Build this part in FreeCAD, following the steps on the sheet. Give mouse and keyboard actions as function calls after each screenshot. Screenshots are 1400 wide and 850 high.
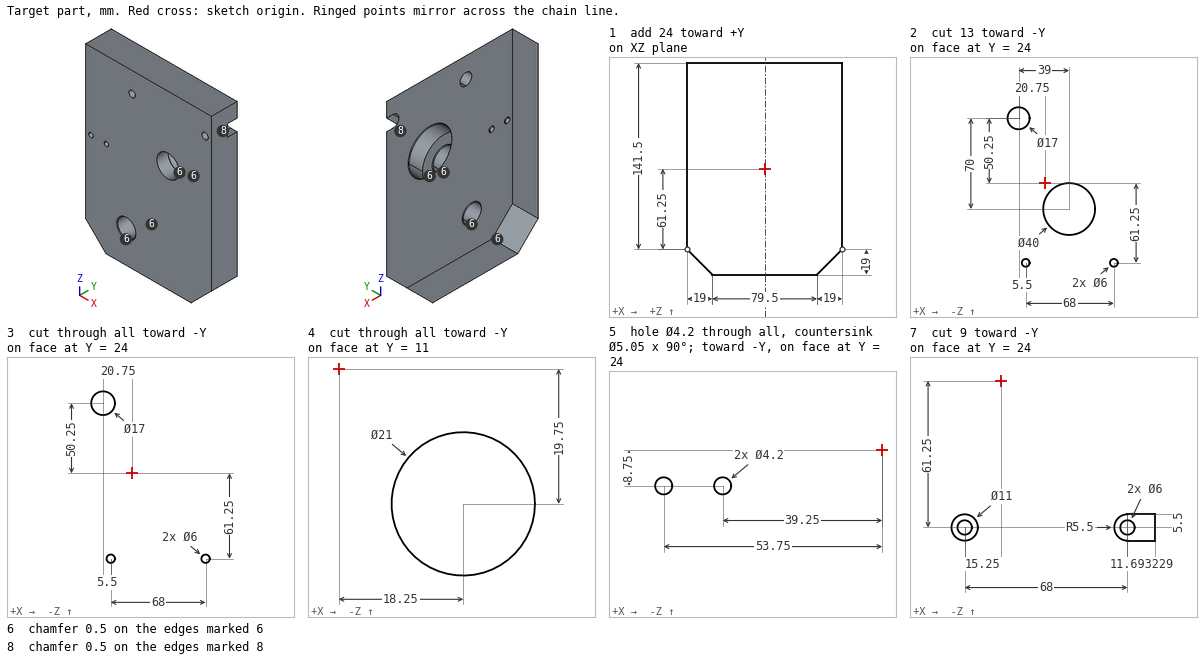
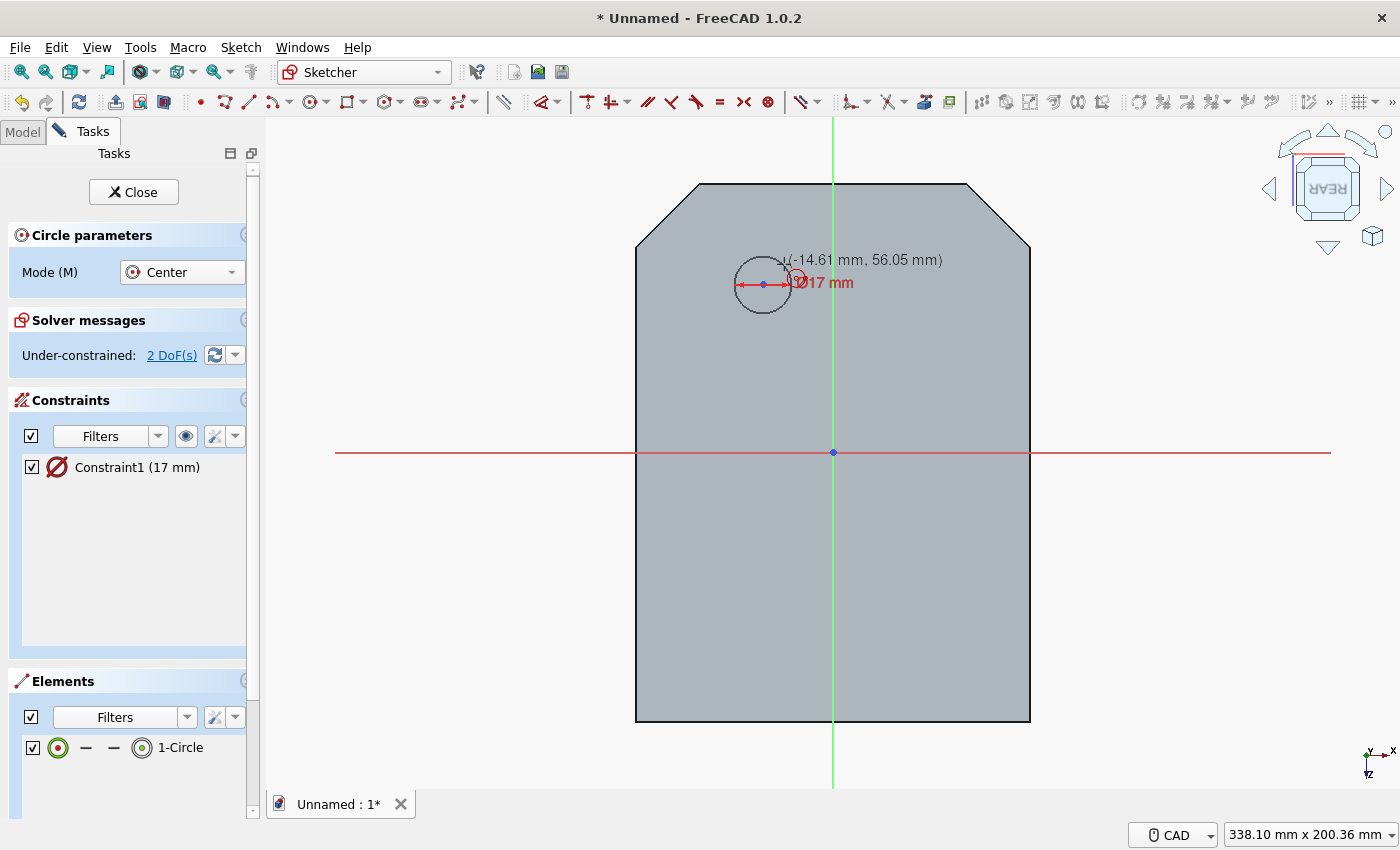
click(894, 519)
move(942, 472)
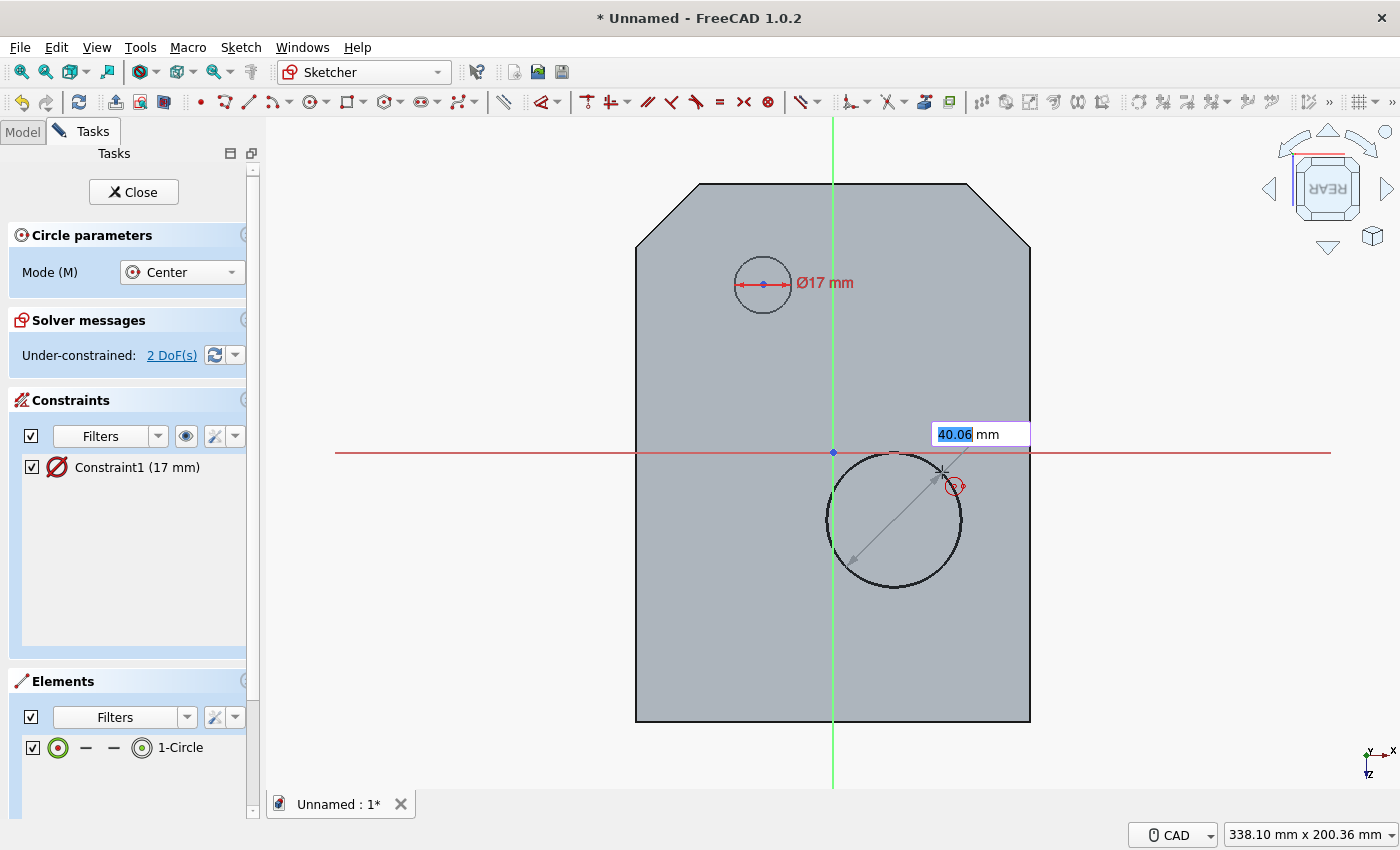
text(40)
key(Return)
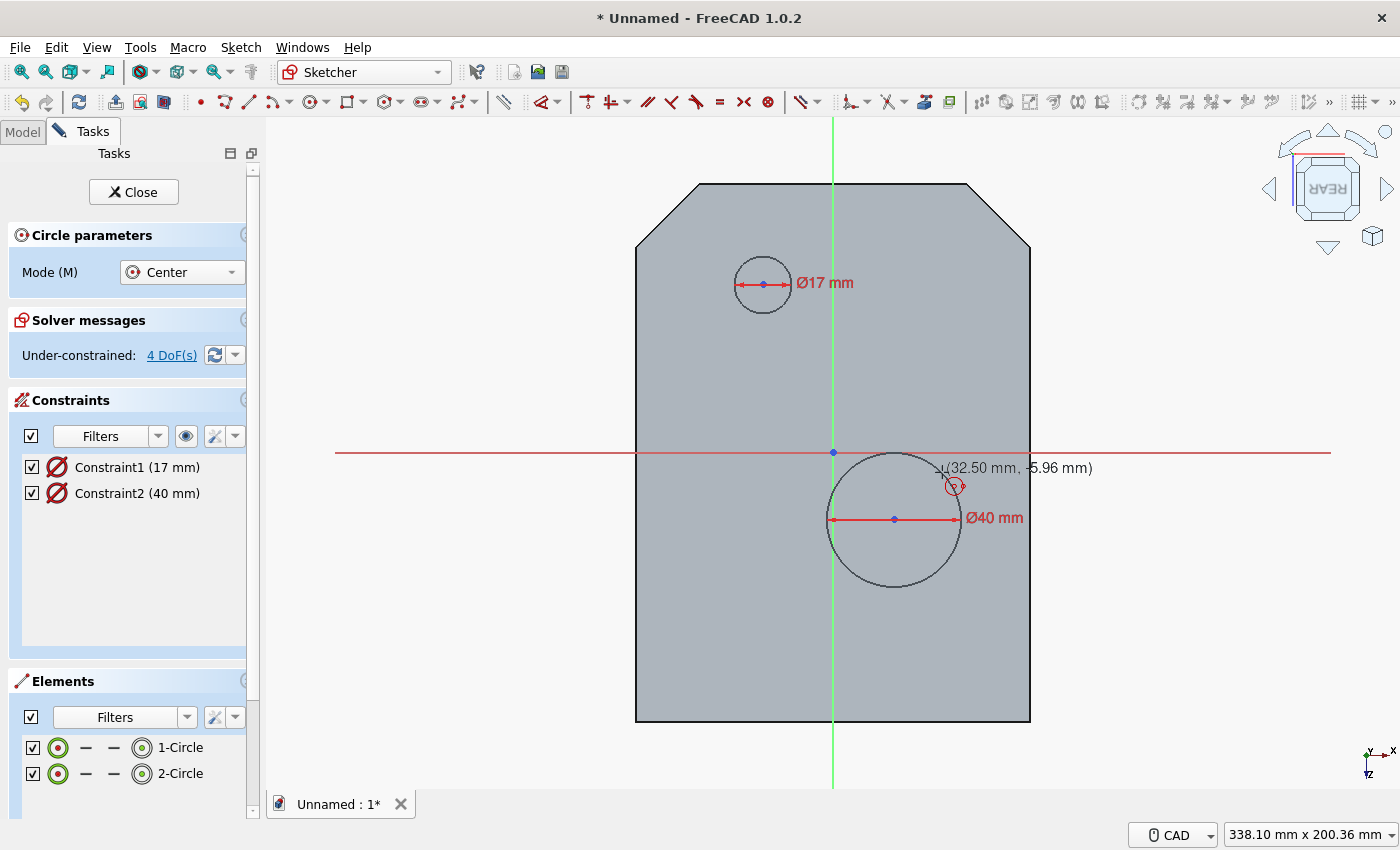
scroll(1010, 658, up, 5)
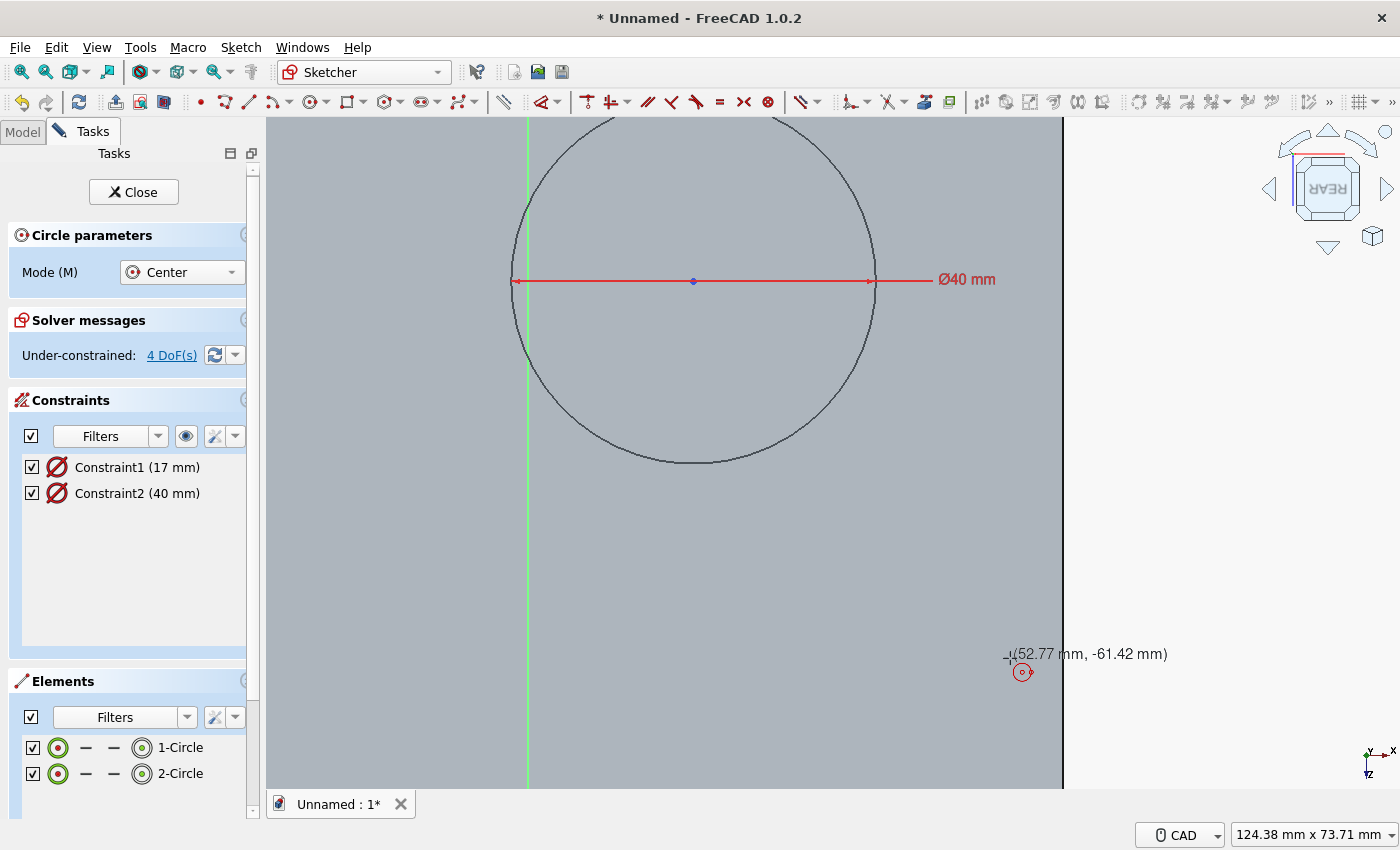
click(1009, 658)
move(1028, 638)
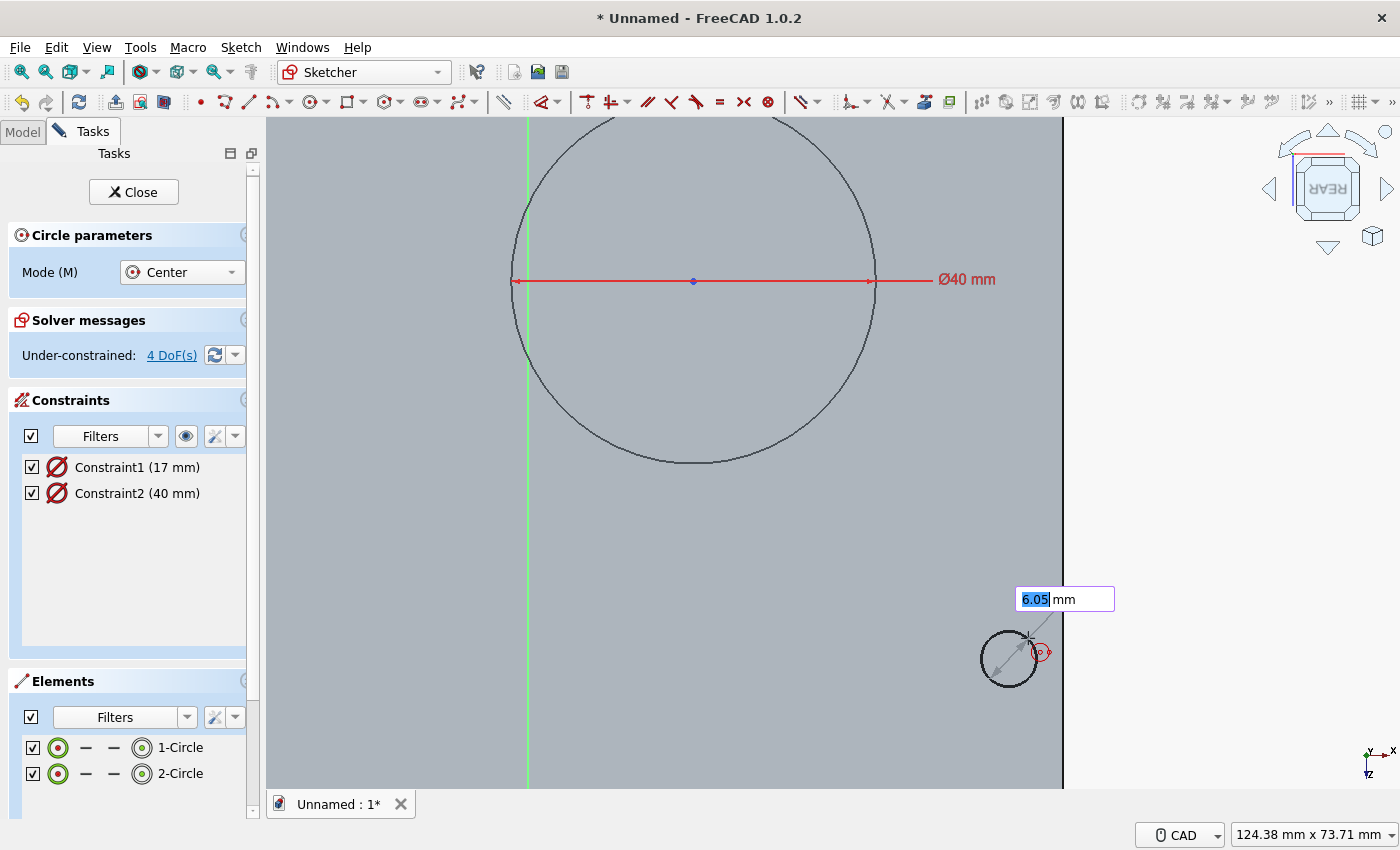
text(6)
key(Return)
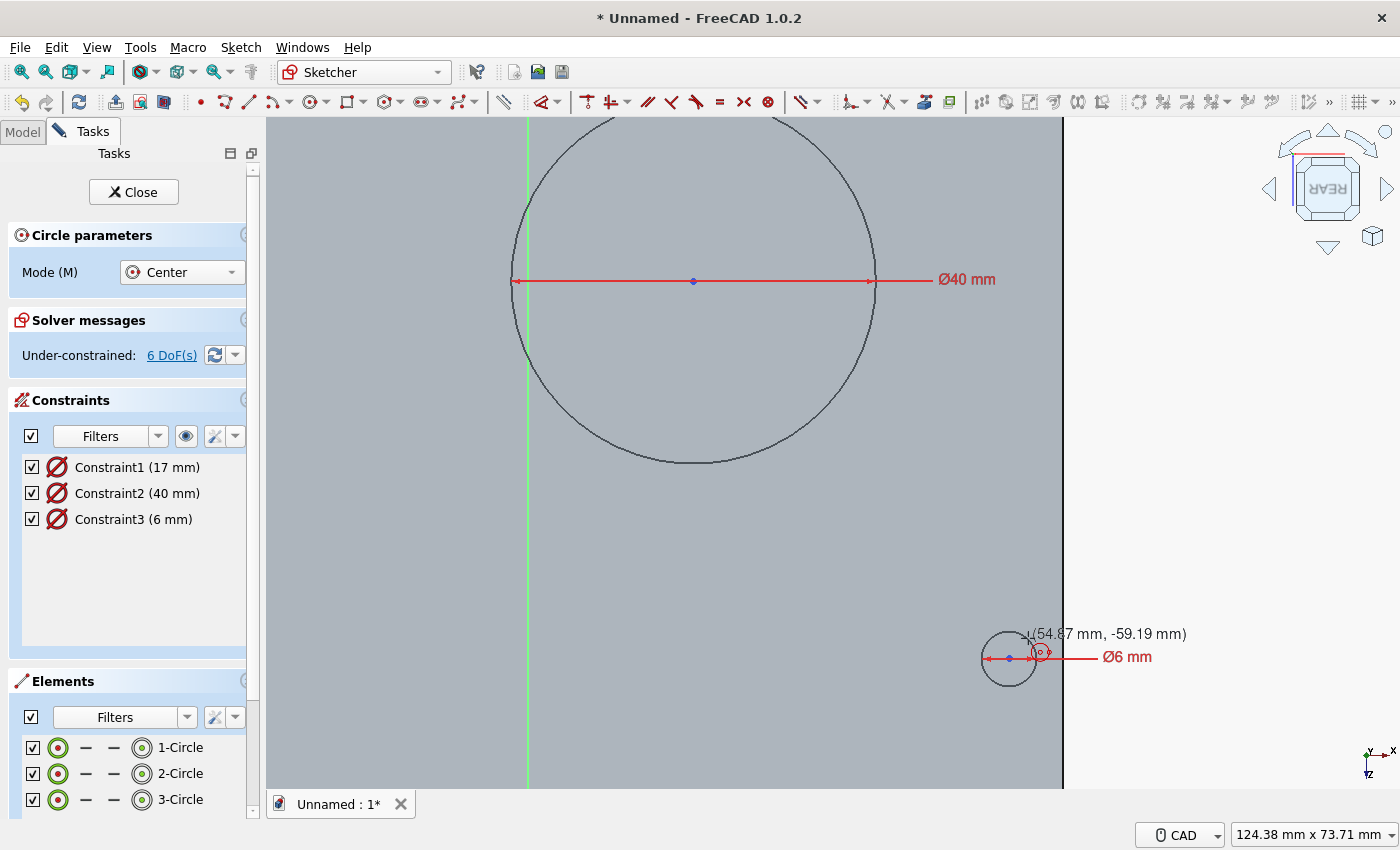
click(389, 658)
move(408, 638)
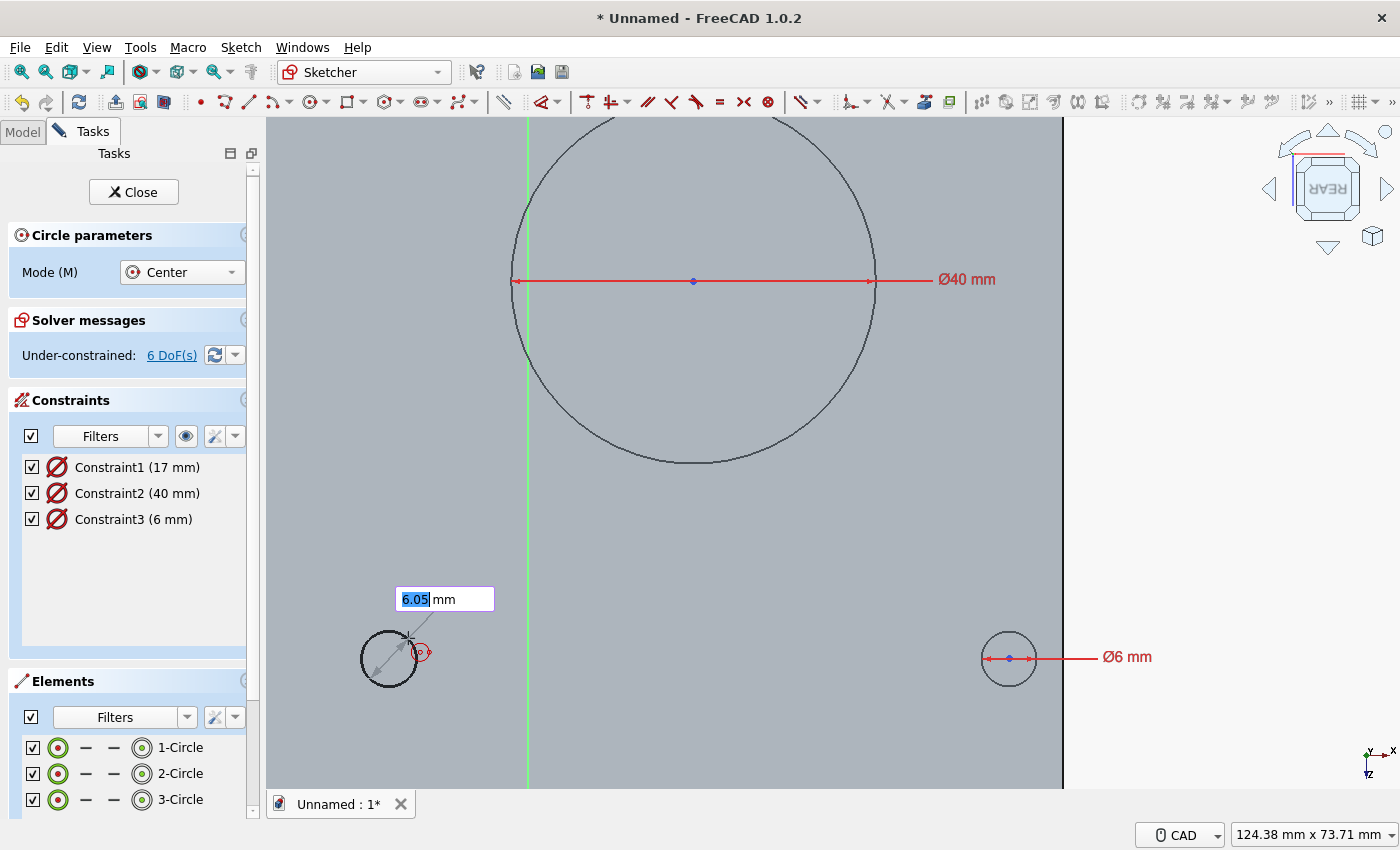
text(6)
key(Return)
key(Escape)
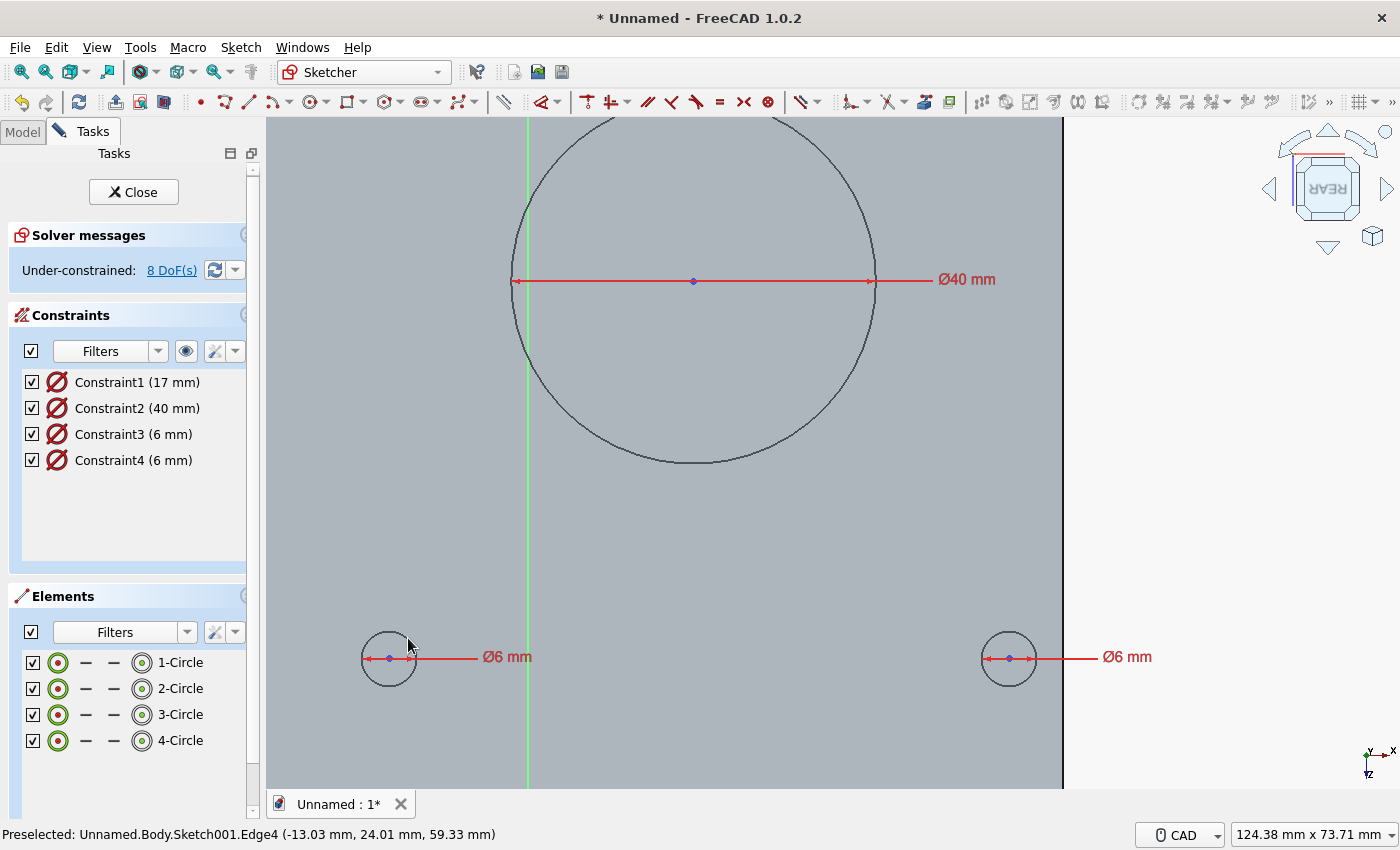
click(1009, 659)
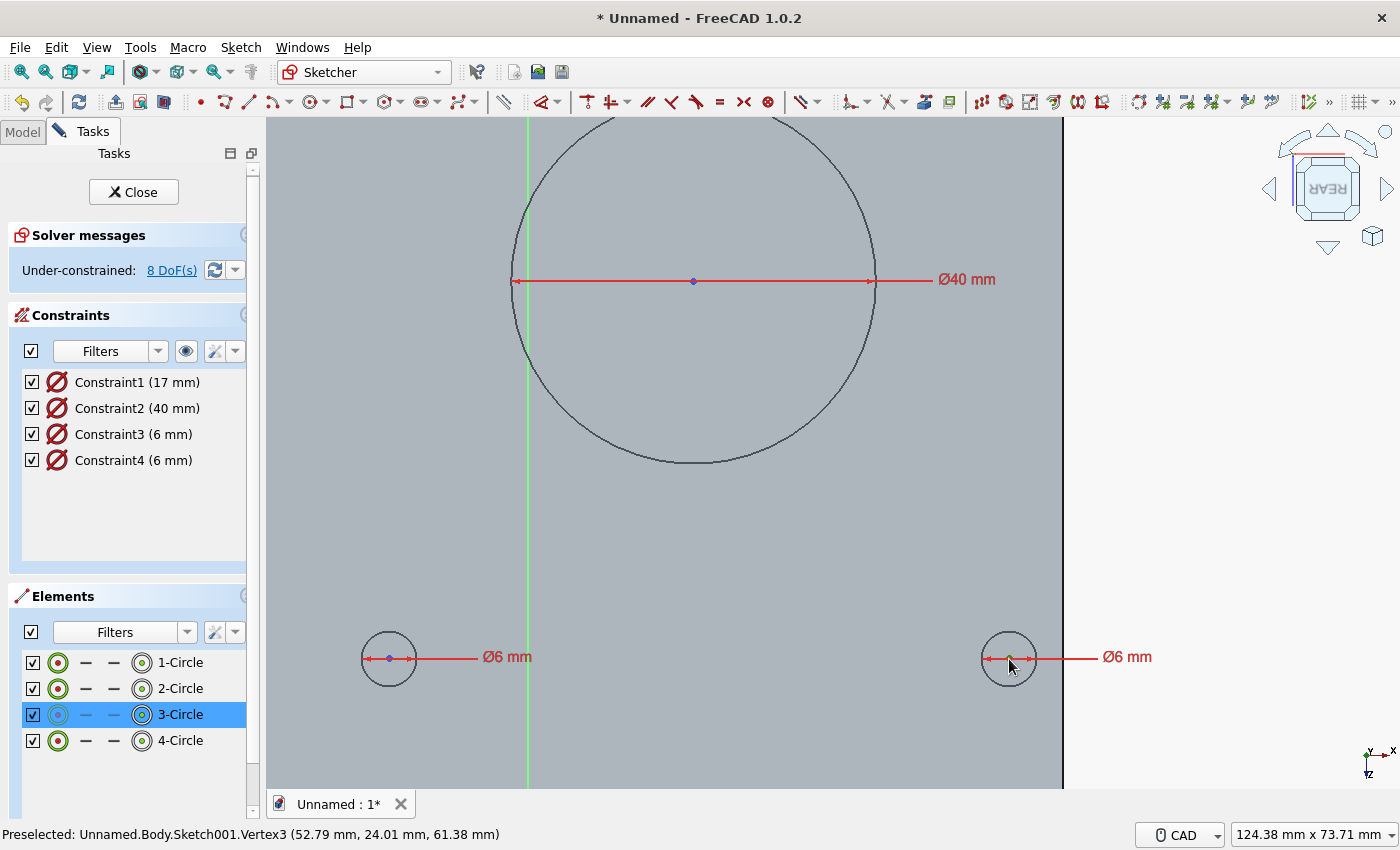
click(389, 659)